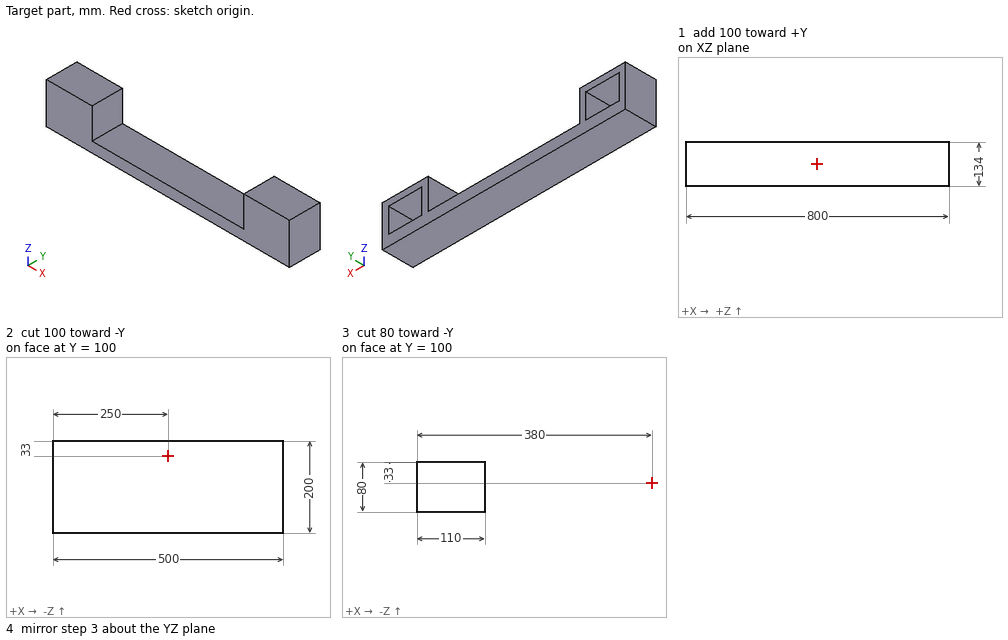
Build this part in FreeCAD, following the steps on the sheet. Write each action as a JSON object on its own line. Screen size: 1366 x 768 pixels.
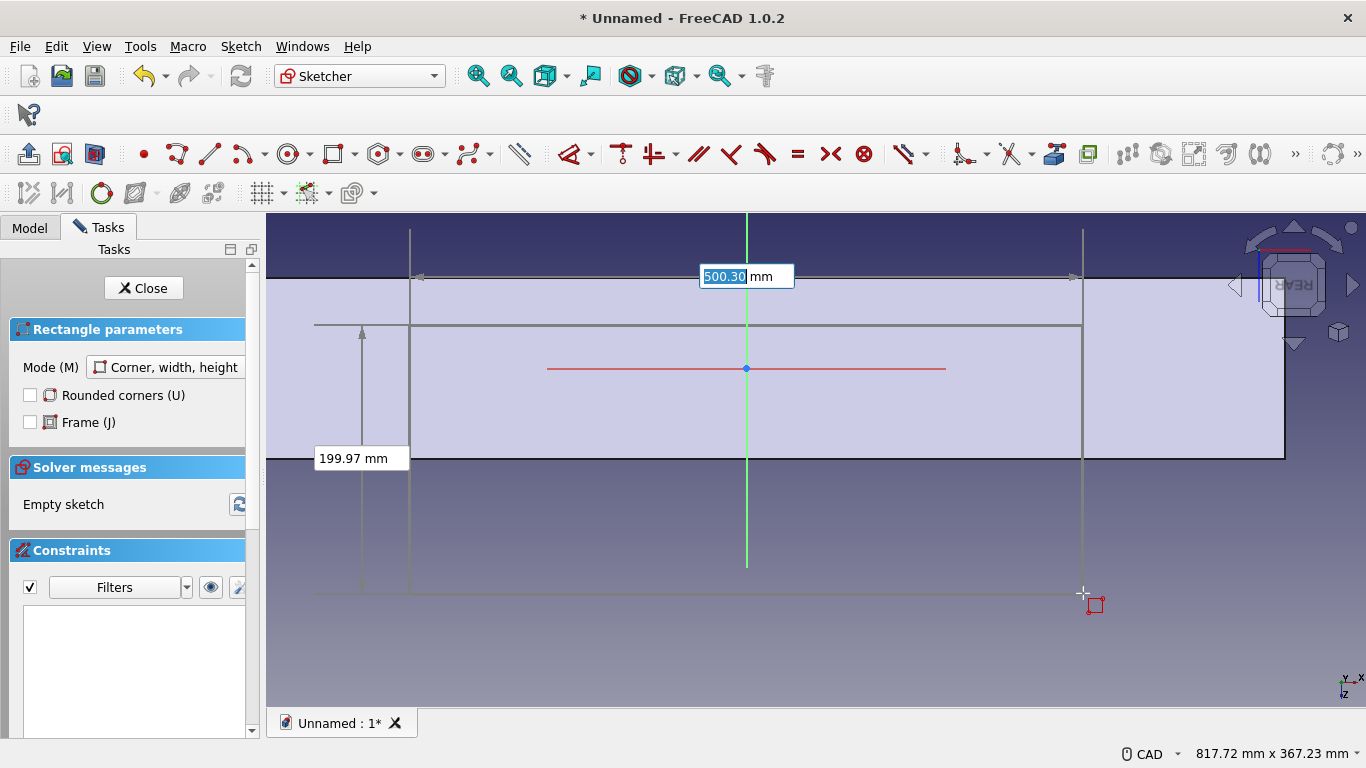
{"action": "type", "text": "500"}
{"action": "key", "text": "Tab"}
{"action": "type", "text": "200"}
{"action": "key", "text": "Return"}
{"action": "key", "text": "Escape"}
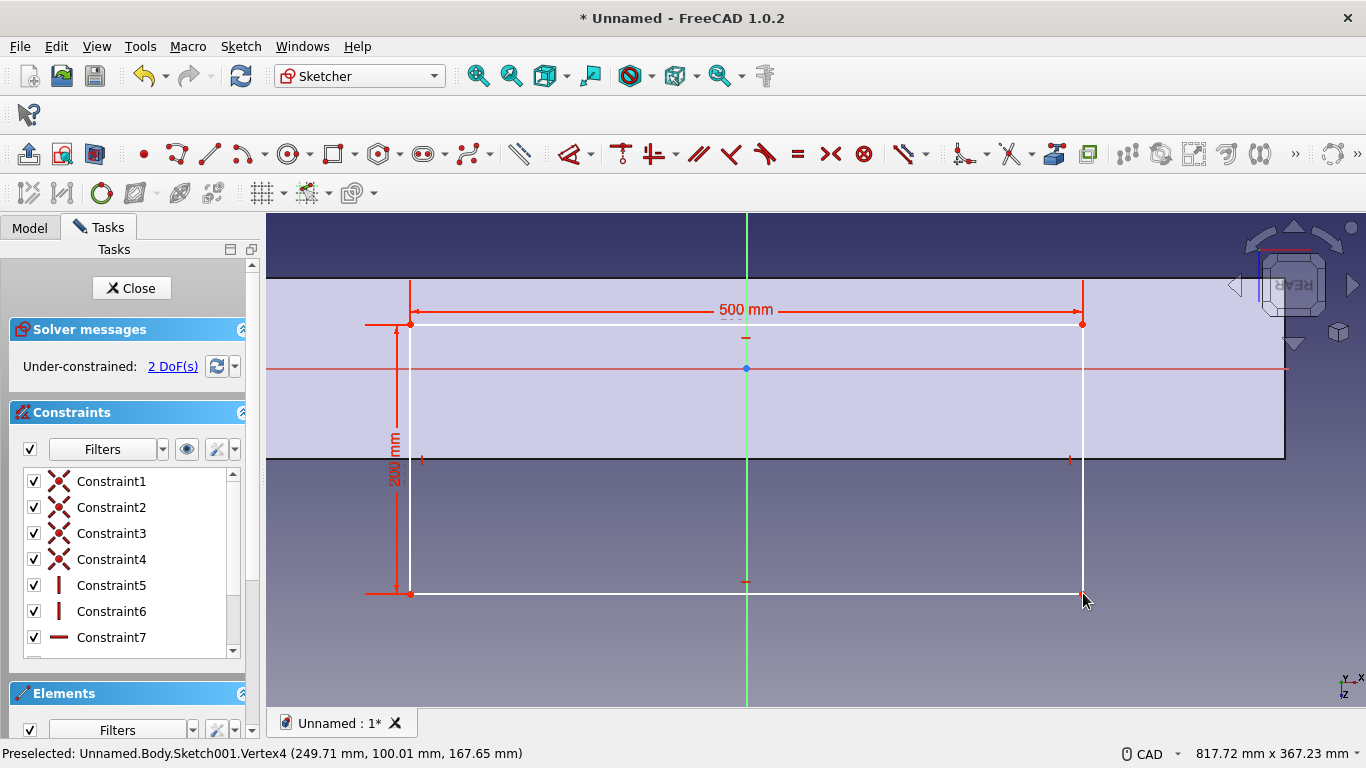
{"action": "key", "text": "d"}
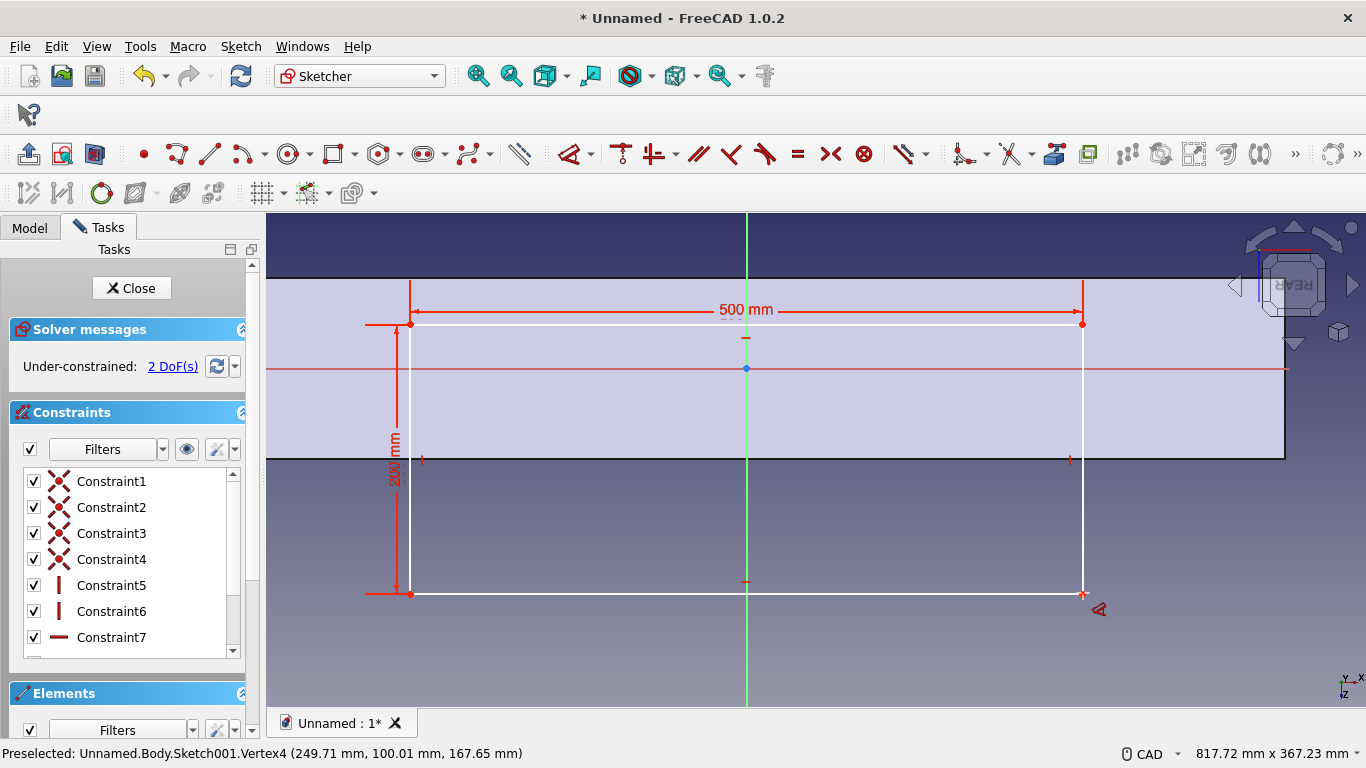
{"action": "left_click", "coordinate": [410, 325]}
{"action": "left_click", "coordinate": [376, 347]}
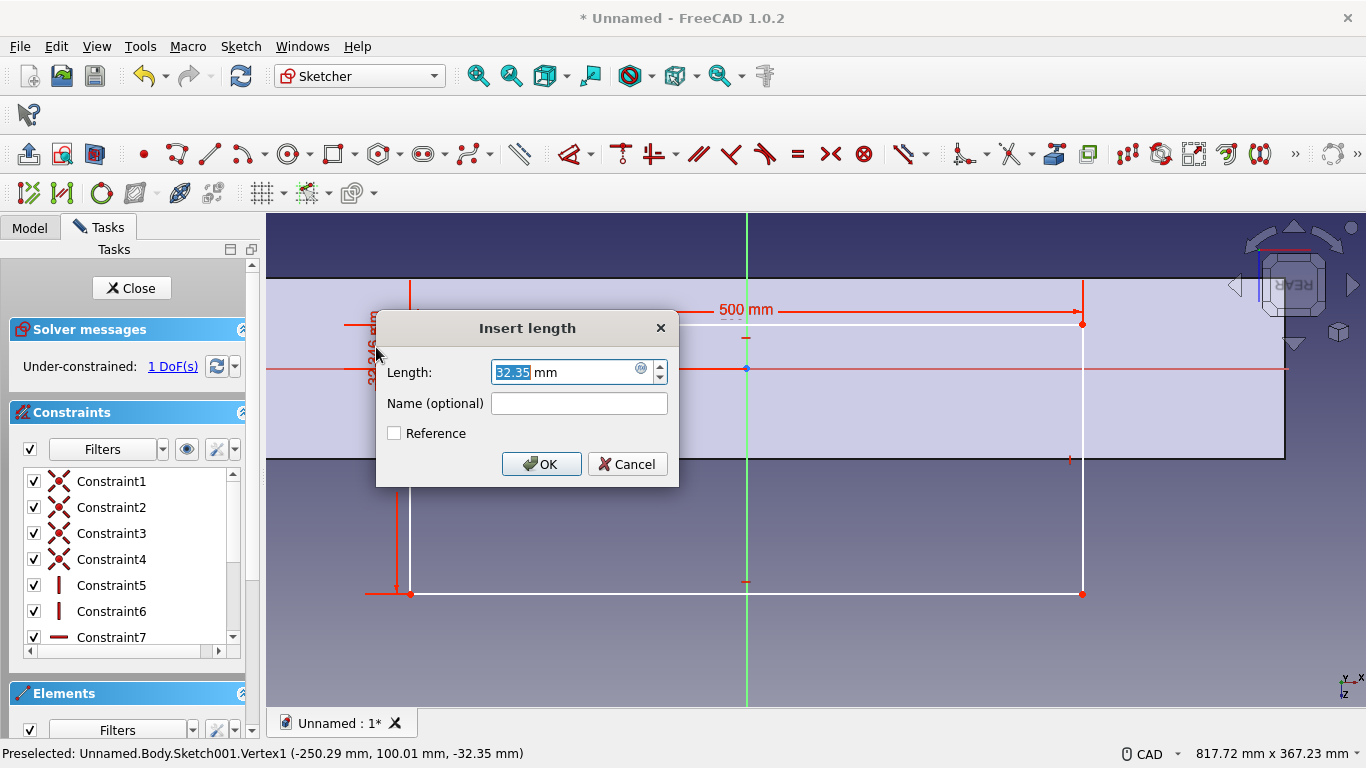
{"action": "type", "text": "33"}
{"action": "key", "text": "Return"}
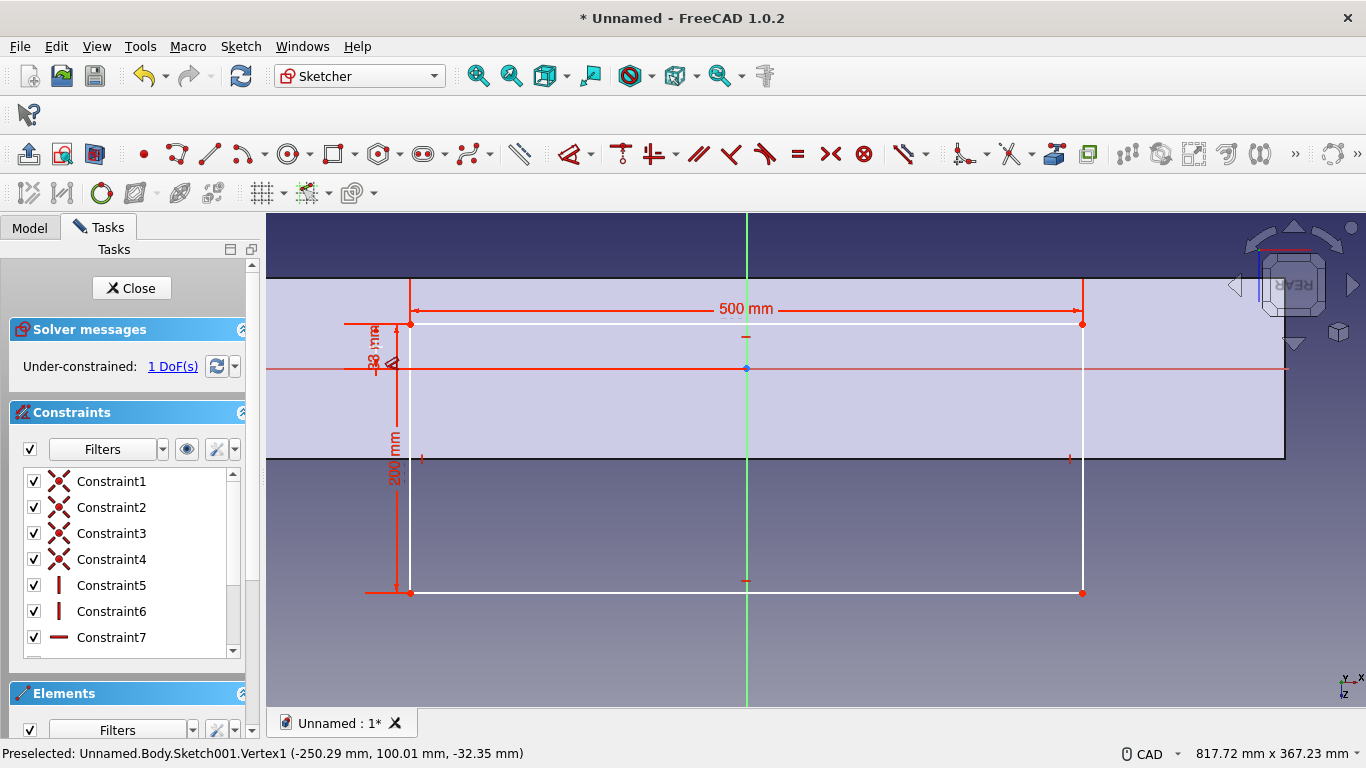
{"action": "left_click", "coordinate": [410, 324]}
{"action": "left_click", "coordinate": [578, 290]}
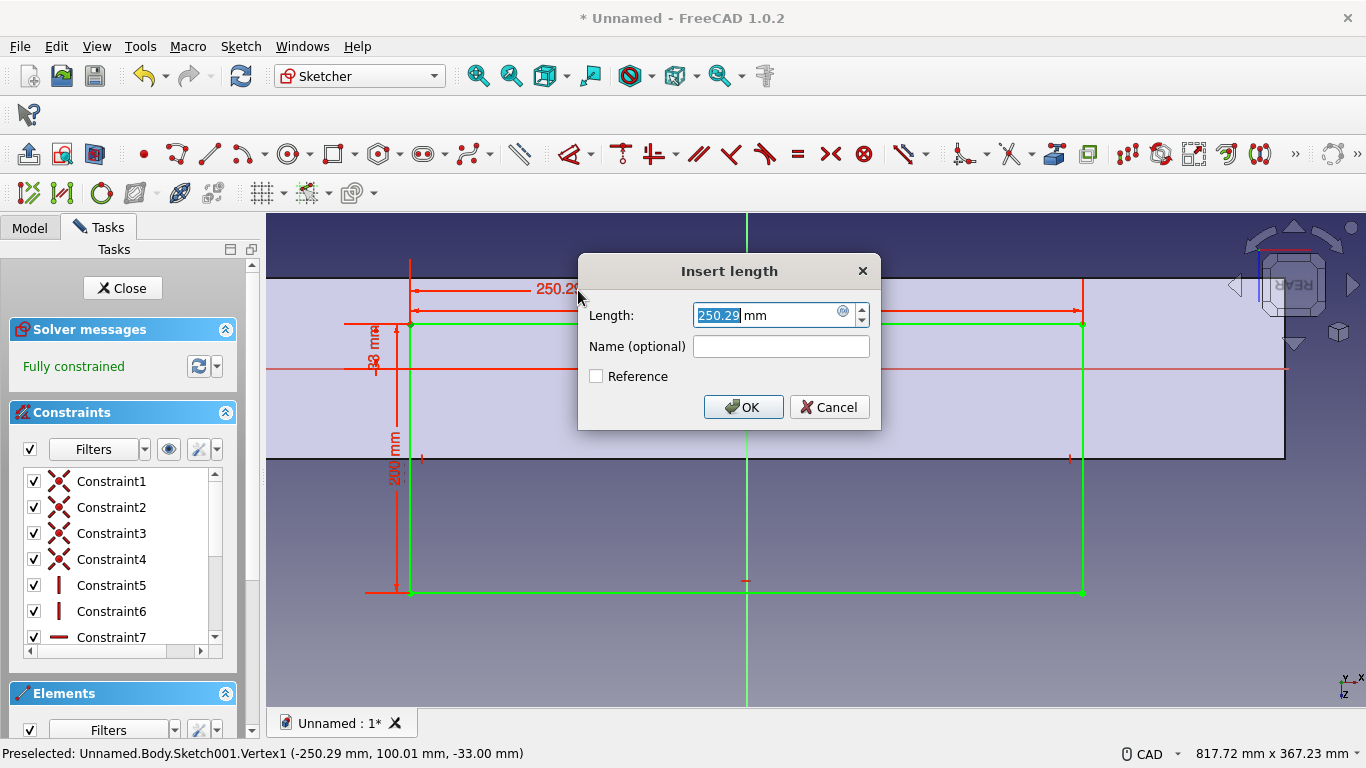
{"action": "type", "text": "250"}
{"action": "key", "text": "Return"}
{"action": "key", "text": "Escape"}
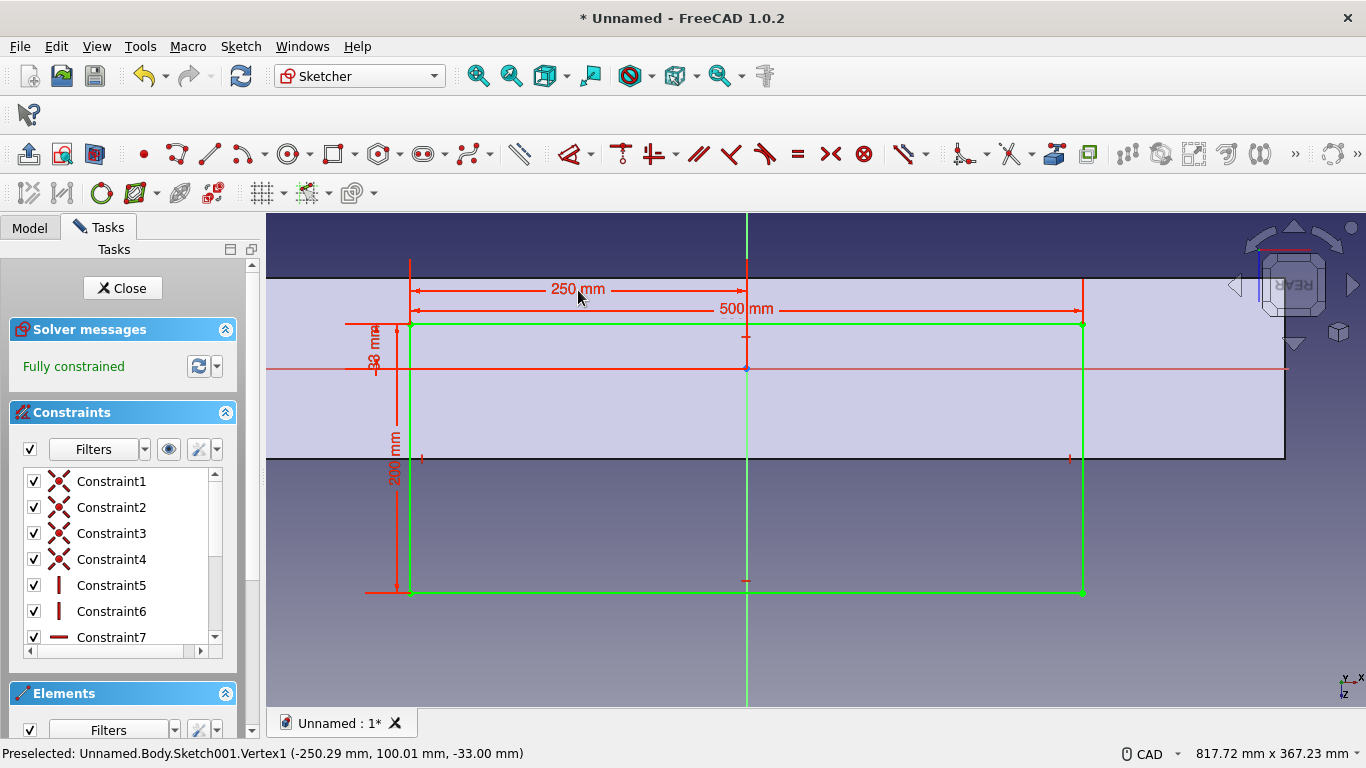
{"action": "left_click", "coordinate": [123, 288]}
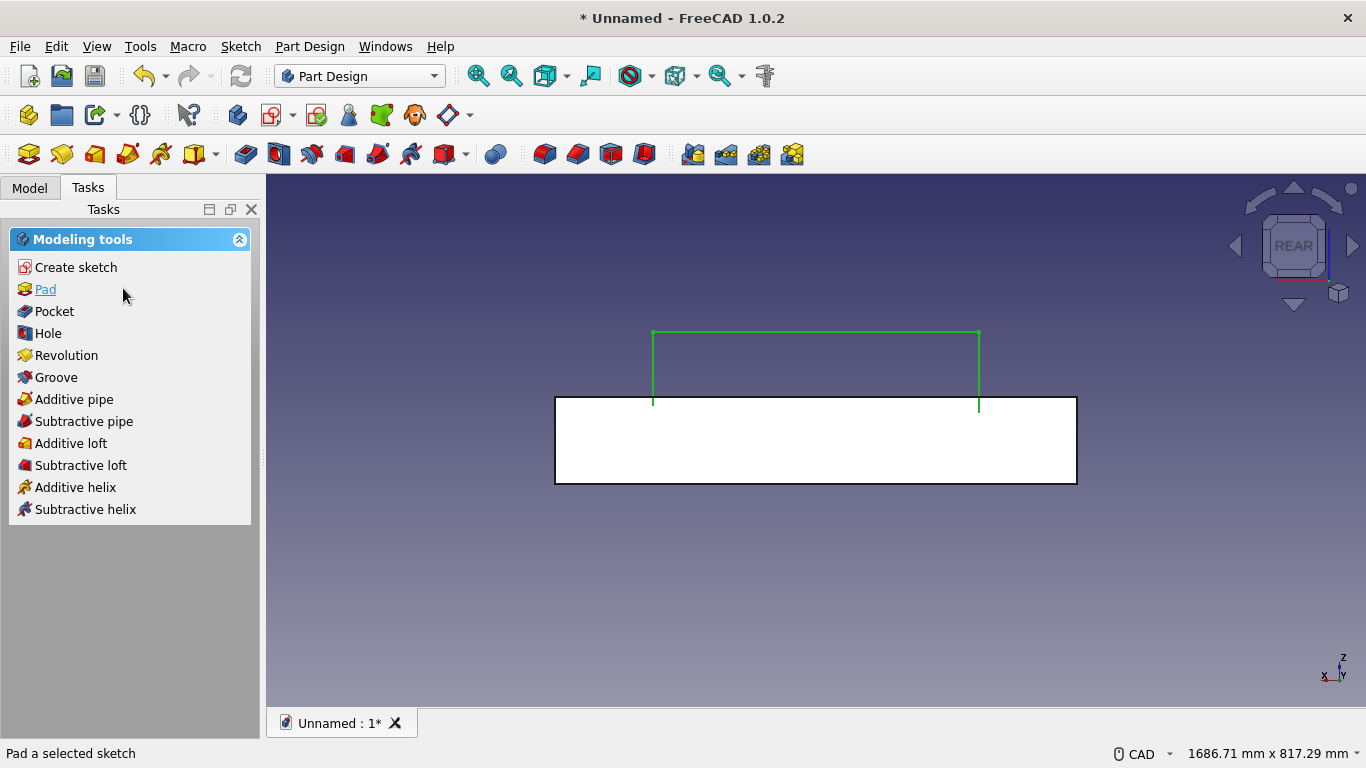
{"action": "left_click", "coordinate": [246, 154]}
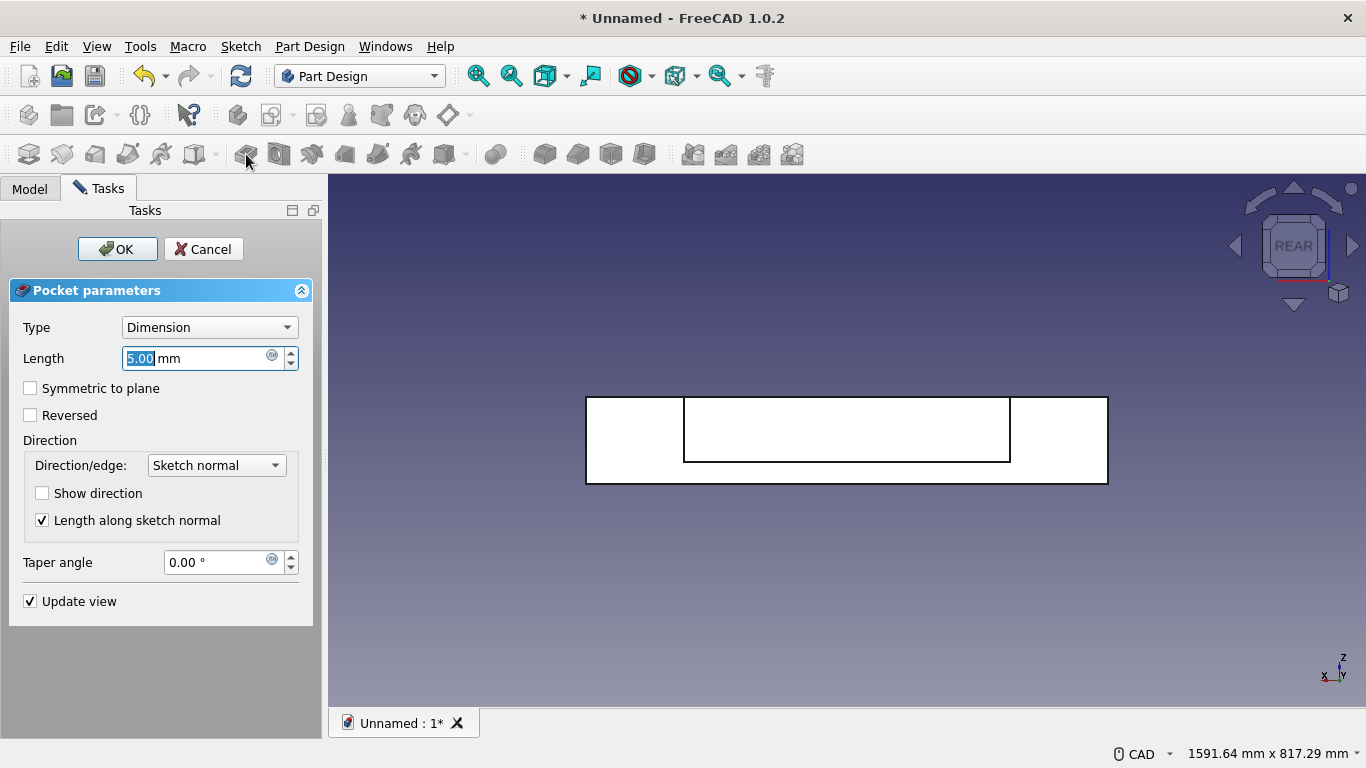
{"action": "type", "text": "100"}
{"action": "key", "text": "Tab"}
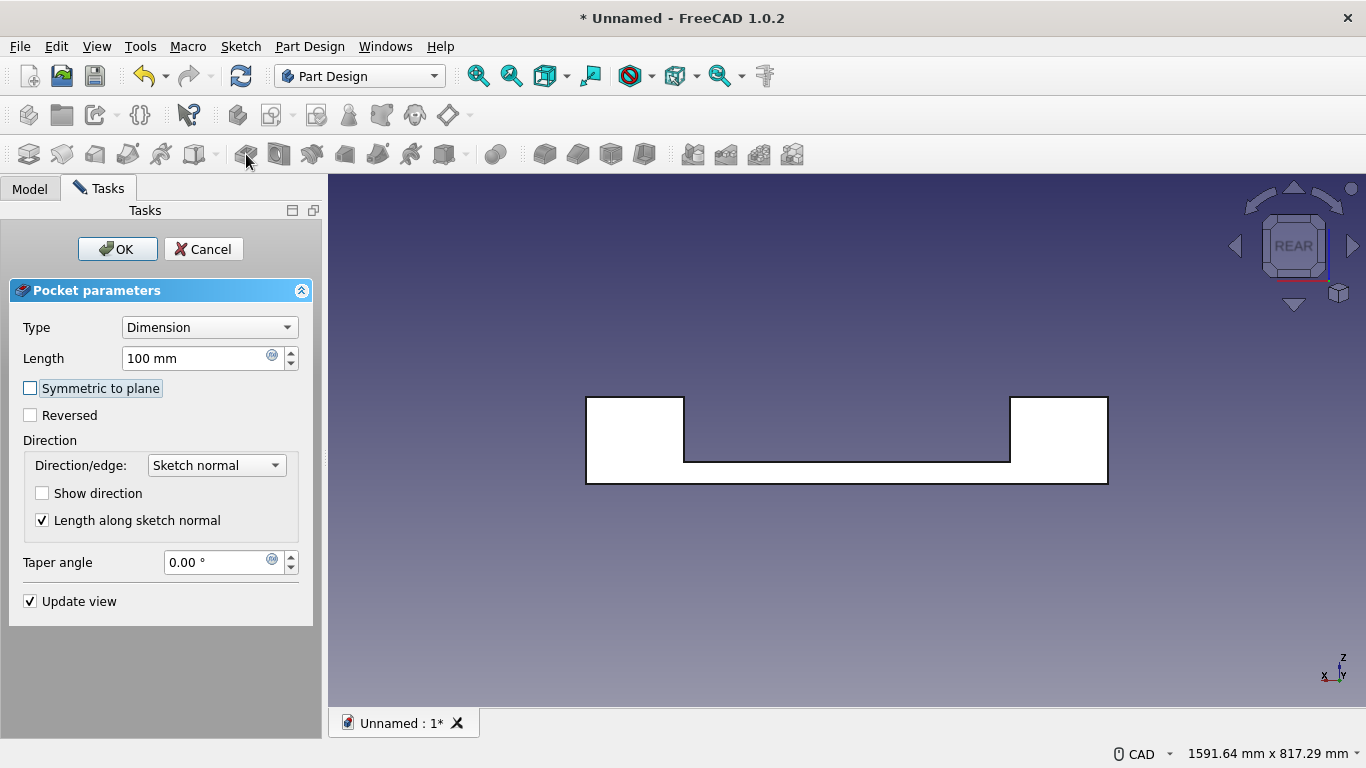
{"action": "left_click", "coordinate": [118, 249]}